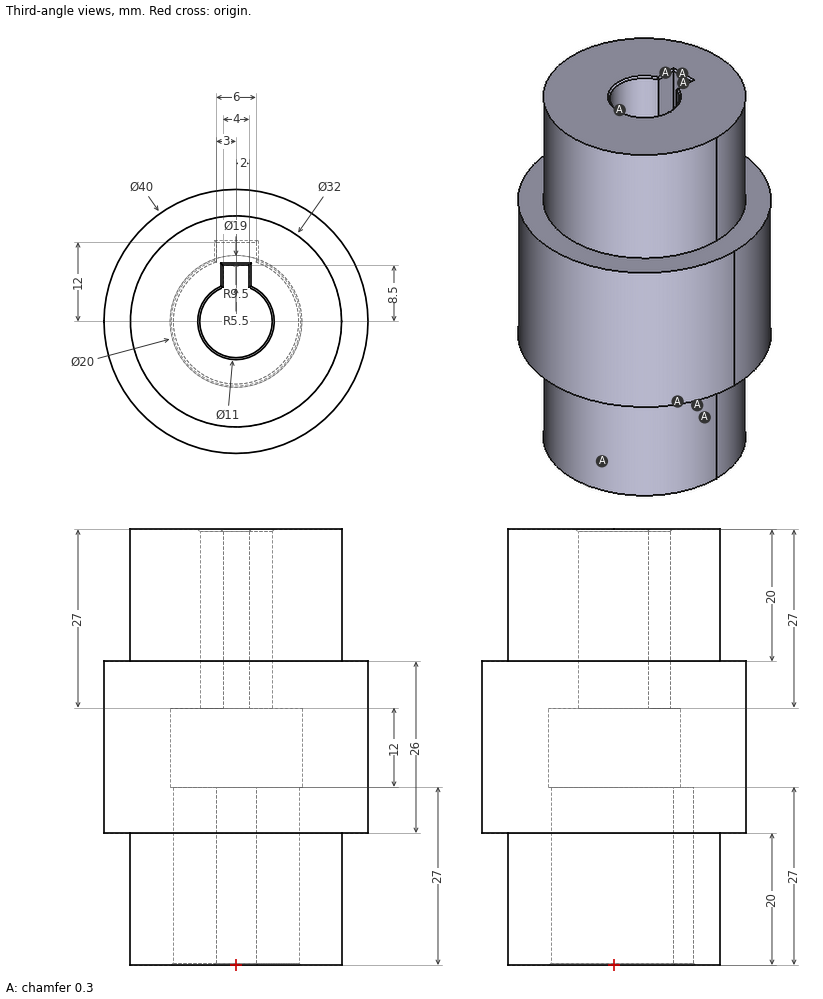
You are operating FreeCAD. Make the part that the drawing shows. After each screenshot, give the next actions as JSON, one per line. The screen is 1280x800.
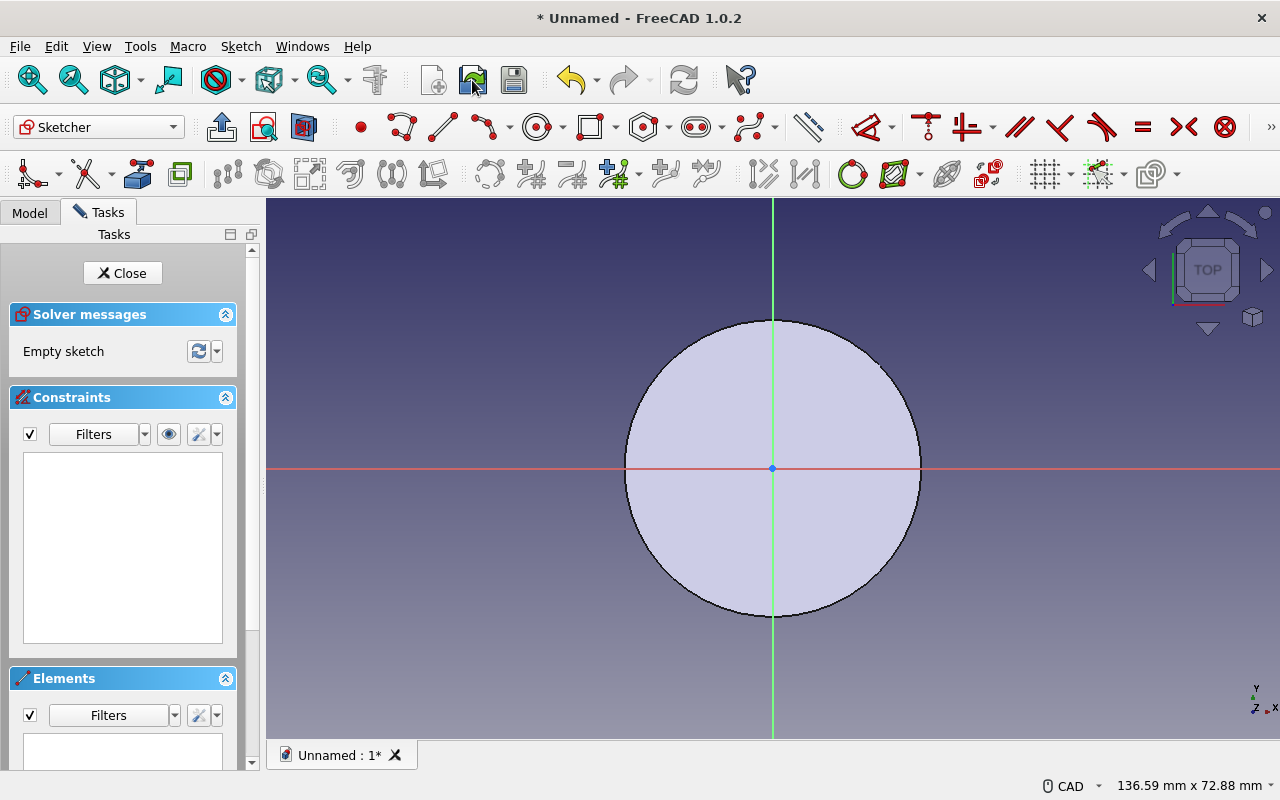
{"action": "scroll", "coordinate": [912, 469], "scroll_direction": "up", "scroll_amount": 2}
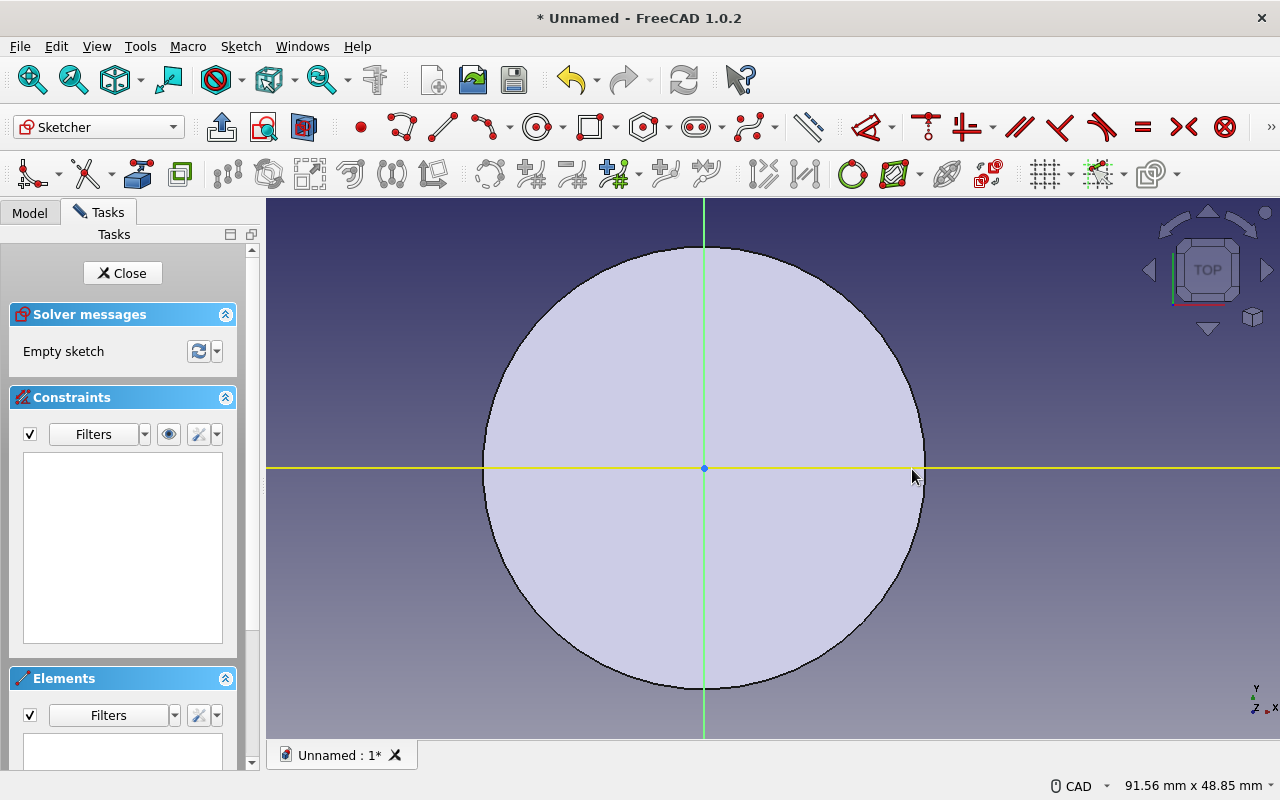
{"action": "left_click", "coordinate": [536, 128]}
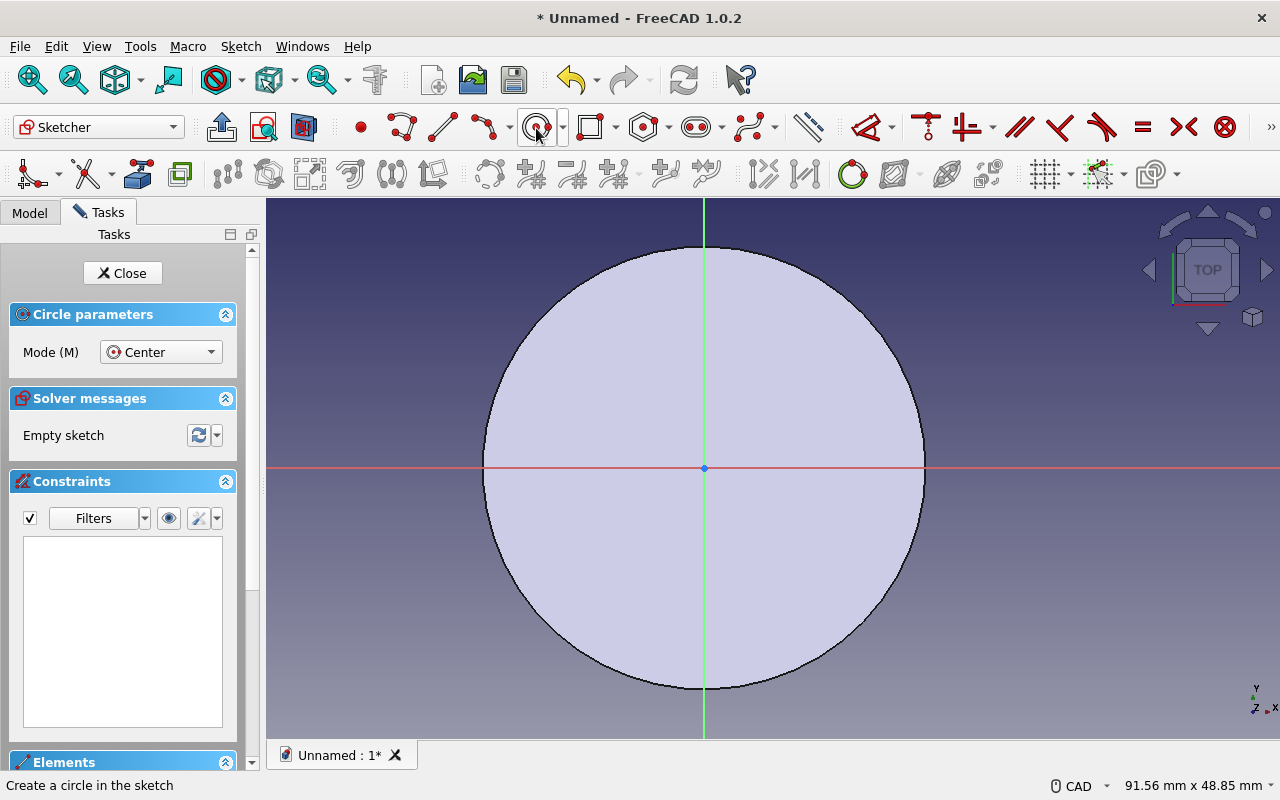
{"action": "left_click", "coordinate": [704, 468]}
{"action": "left_click", "coordinate": [829, 343]}
{"action": "key", "text": "Escape"}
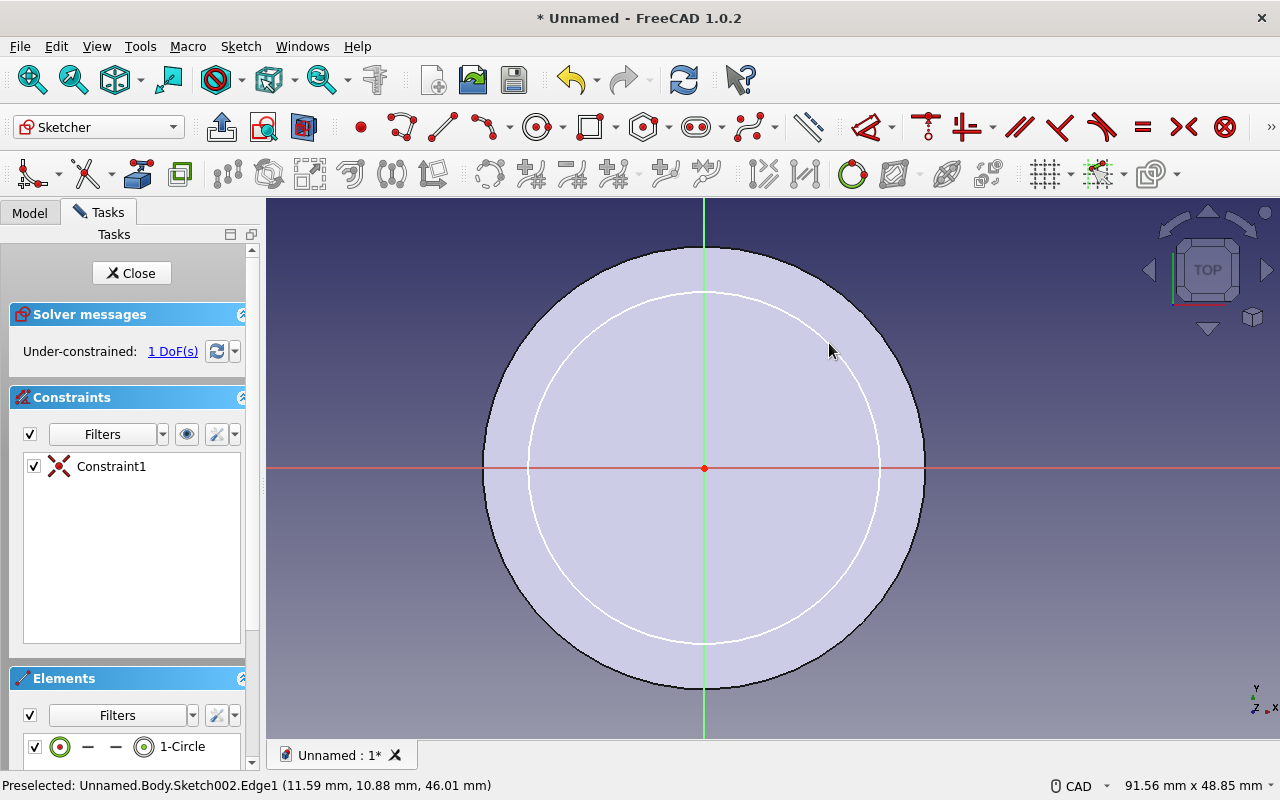
{"action": "left_click", "coordinate": [866, 128]}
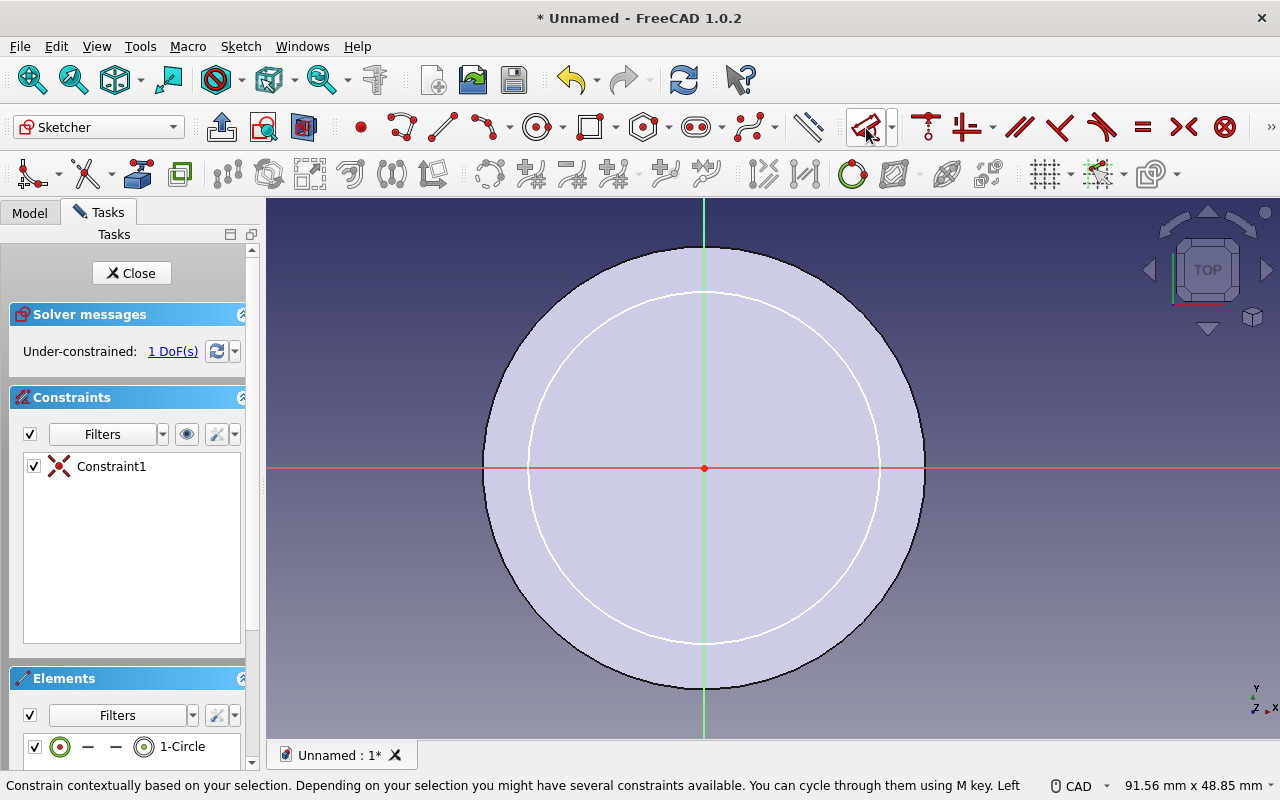
{"action": "left_click", "coordinate": [828, 343]}
{"action": "left_click", "coordinate": [851, 320]}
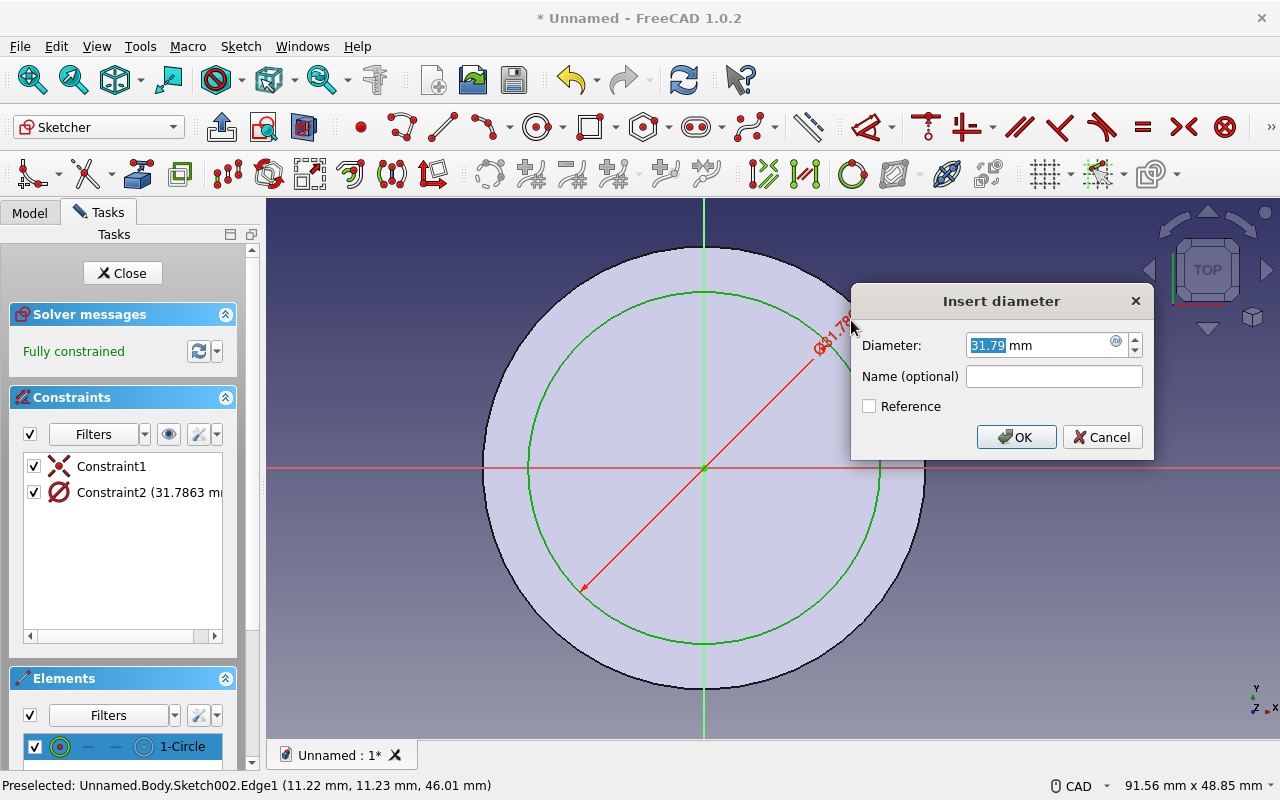
{"action": "type", "text": "32"}
{"action": "key", "text": "Return"}
{"action": "key", "text": "Escape"}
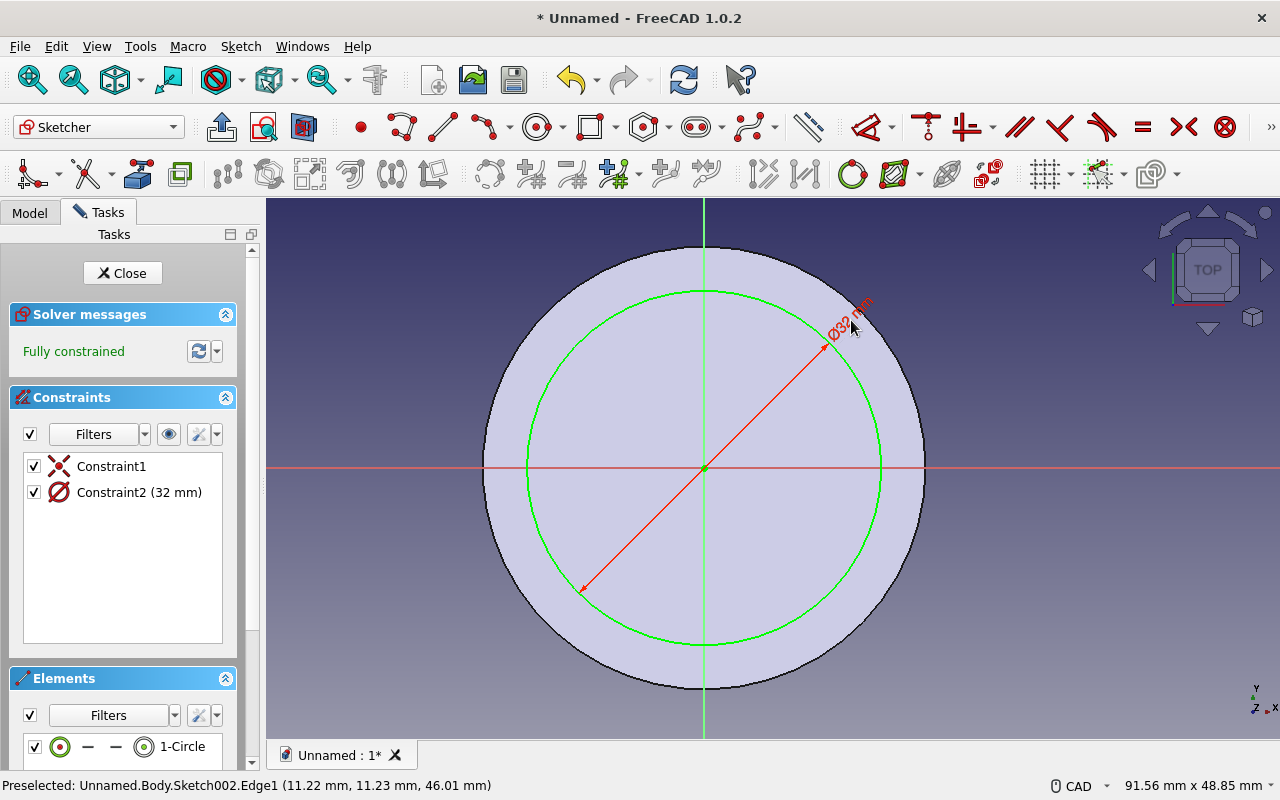
{"action": "left_click", "coordinate": [123, 273]}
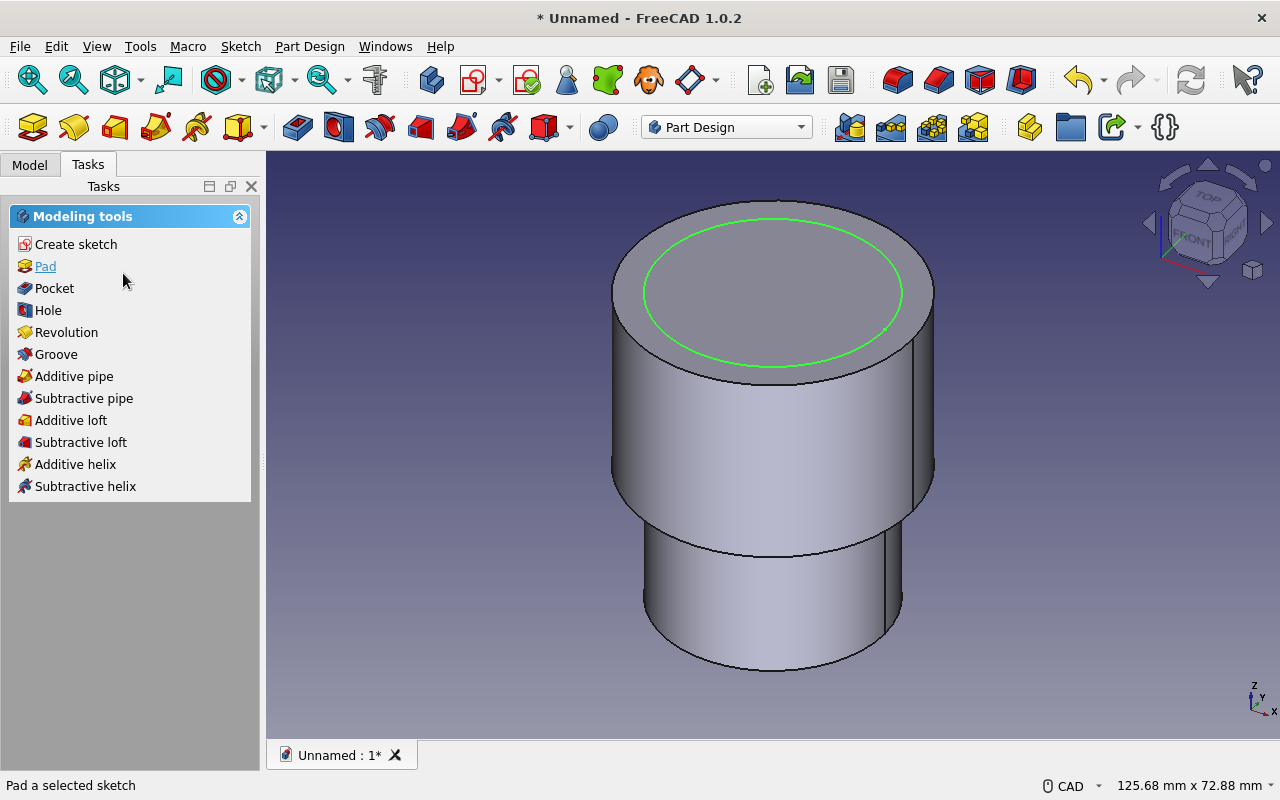
{"action": "left_click", "coordinate": [33, 128]}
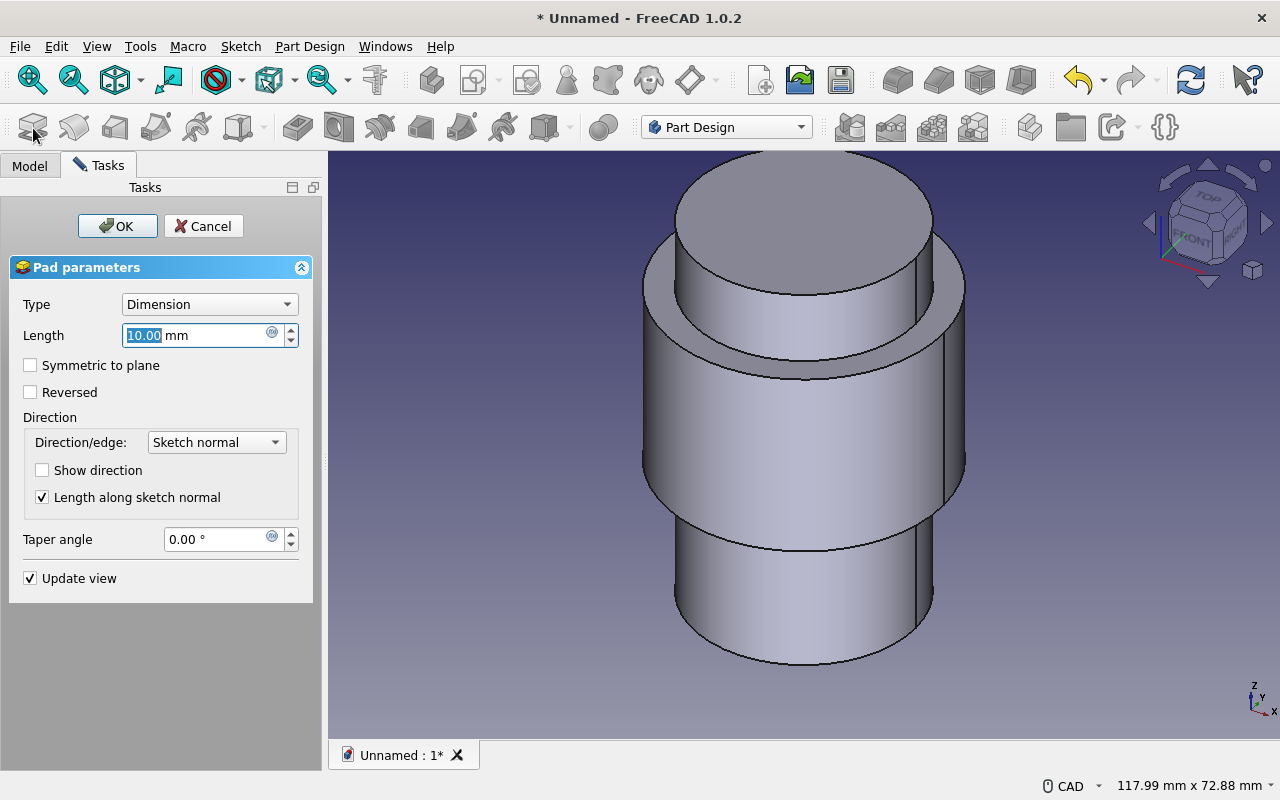
{"action": "type", "text": "20"}
{"action": "key", "text": "Tab"}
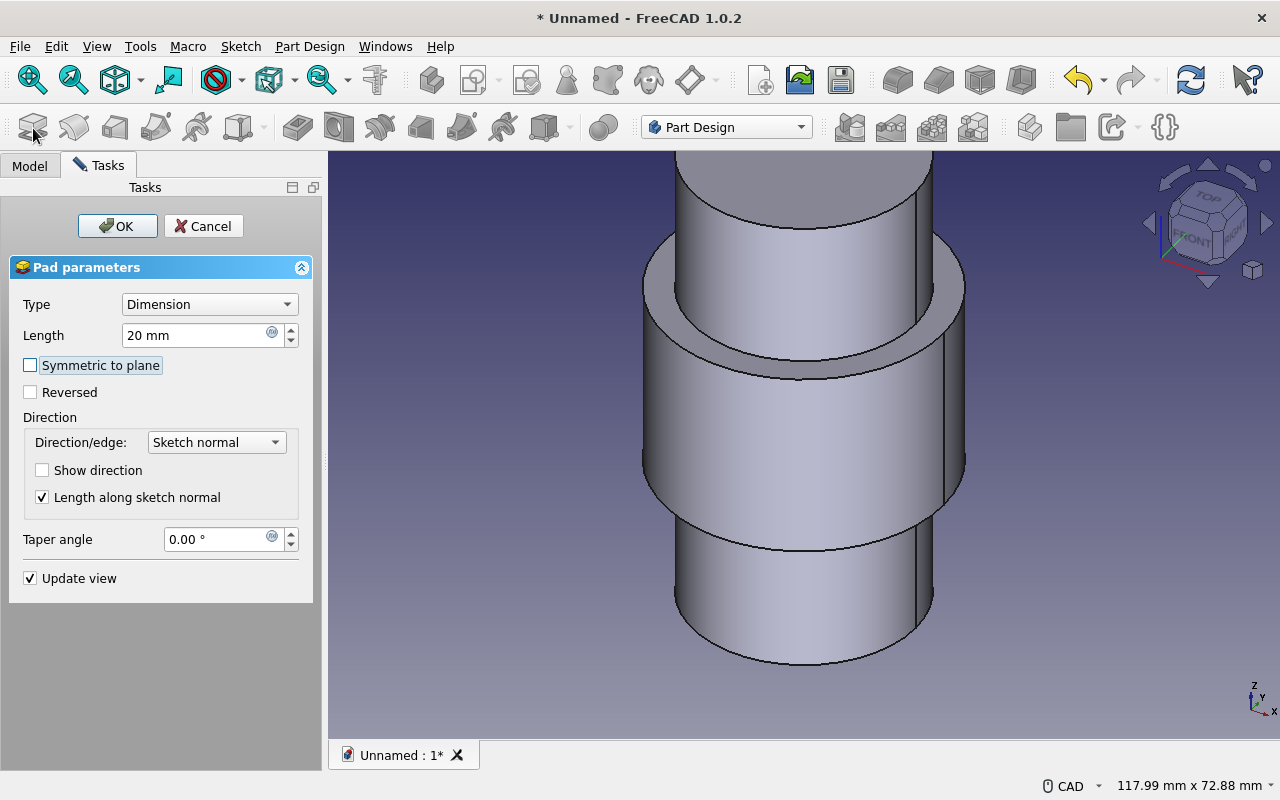
{"action": "left_click", "coordinate": [118, 226]}